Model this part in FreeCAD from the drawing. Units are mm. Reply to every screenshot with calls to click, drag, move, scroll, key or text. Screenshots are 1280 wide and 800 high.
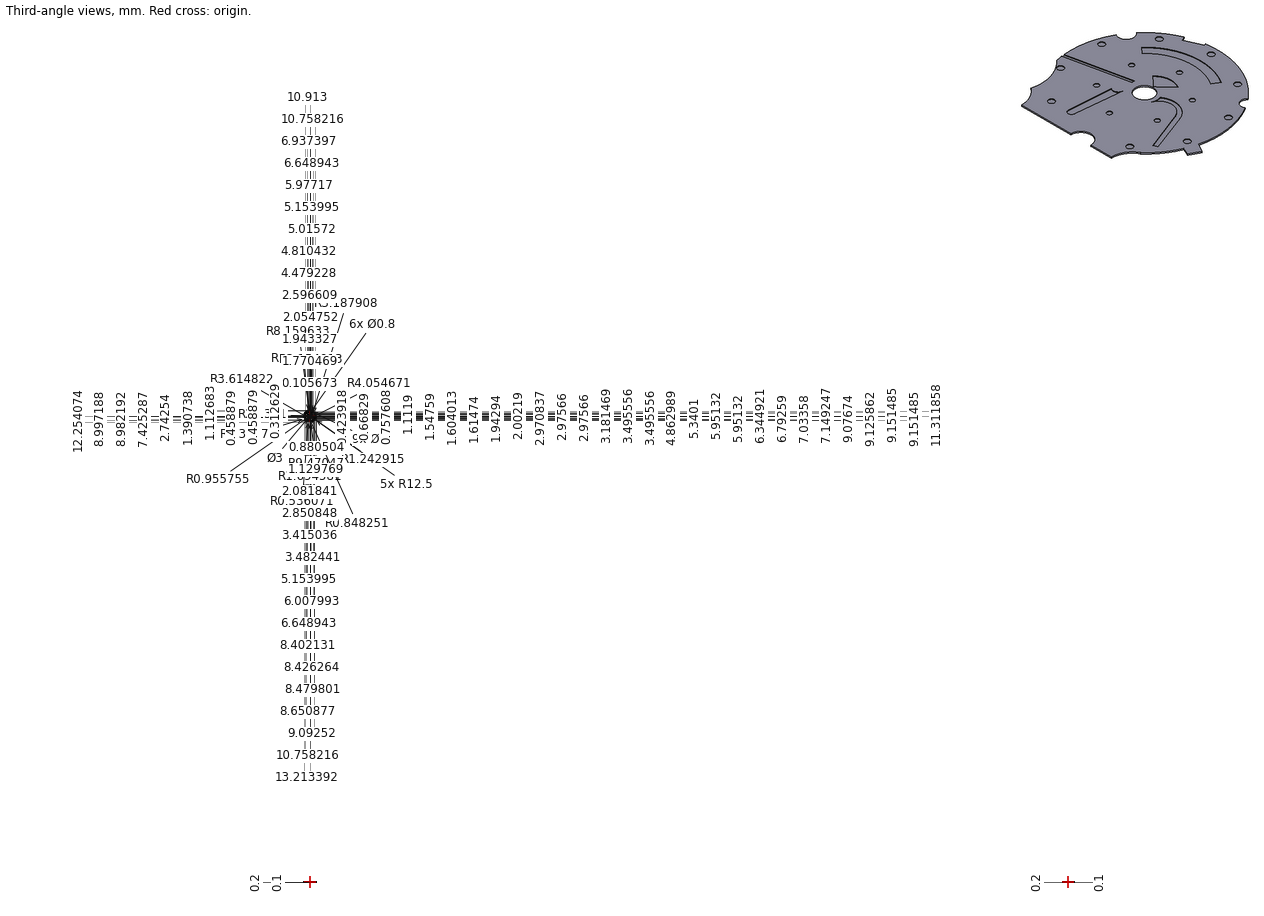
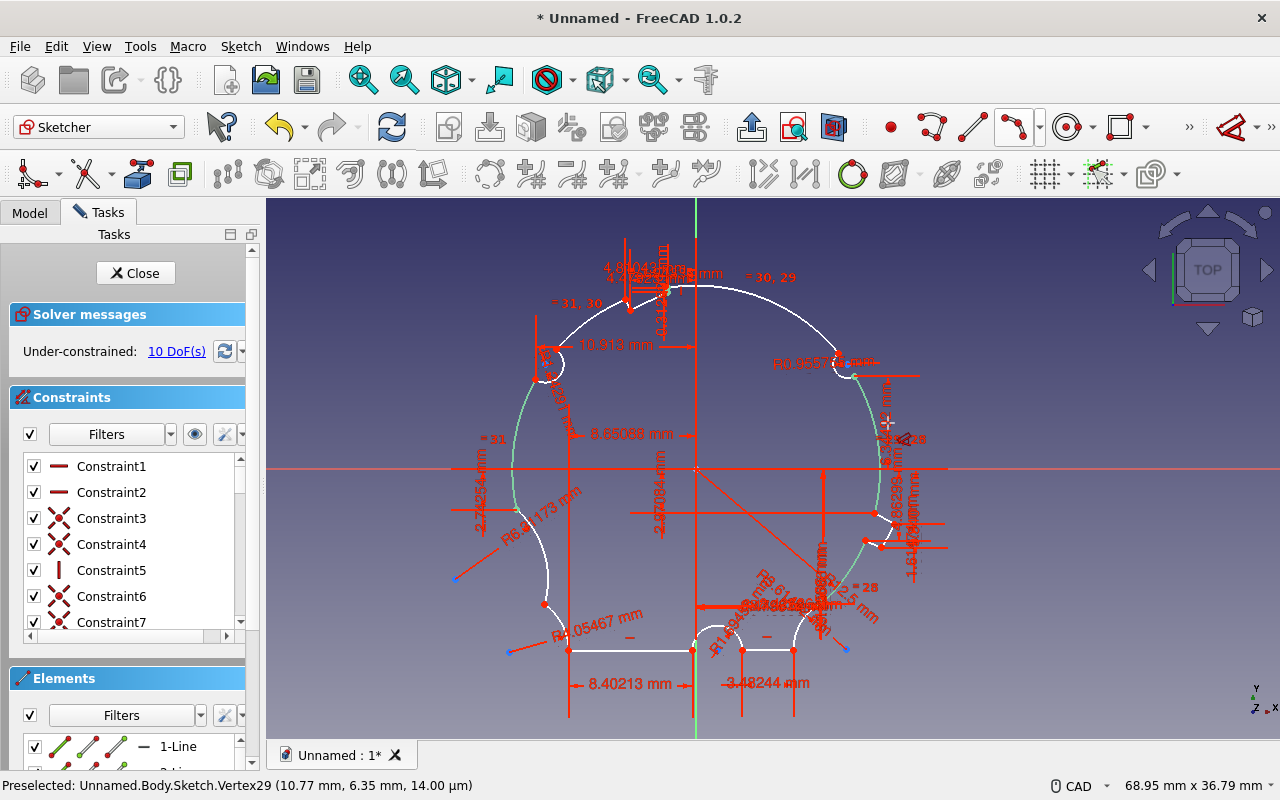
click(545, 604)
click(511, 568)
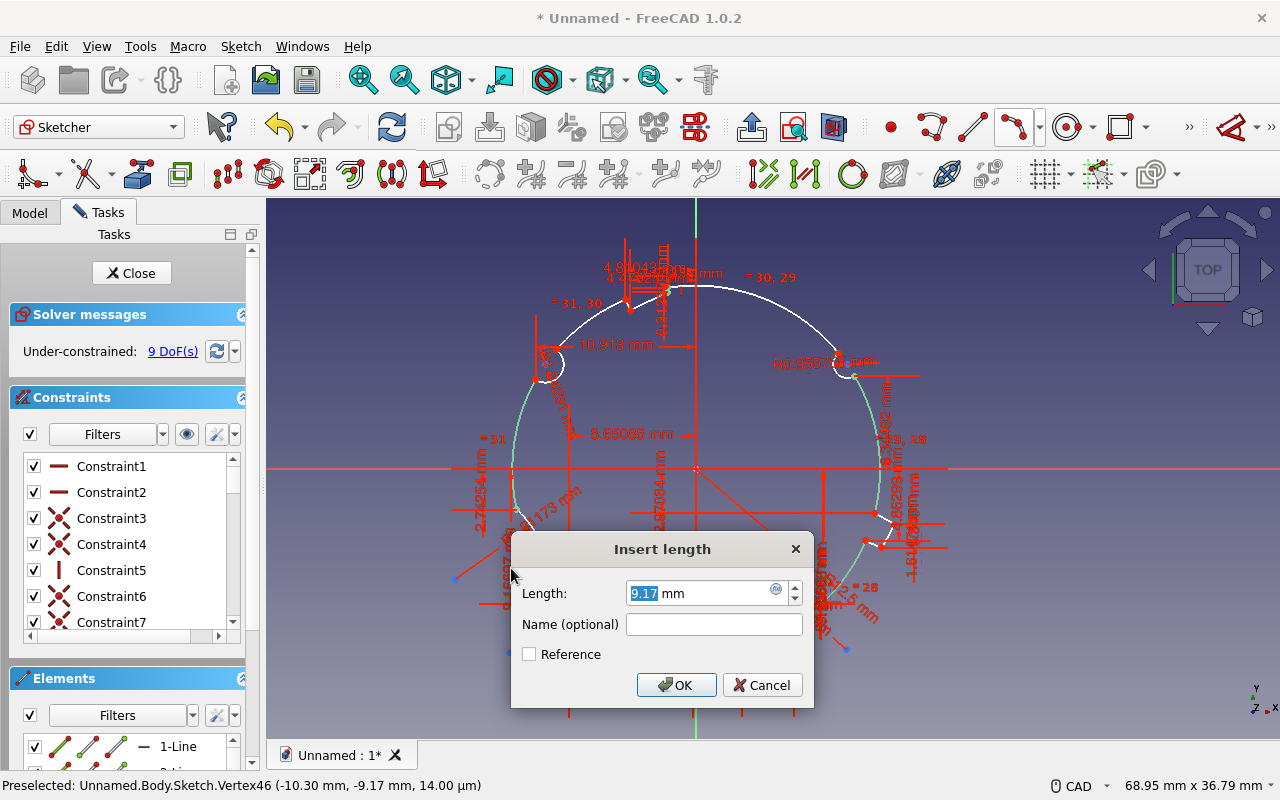
text(8.982192)
key(Return)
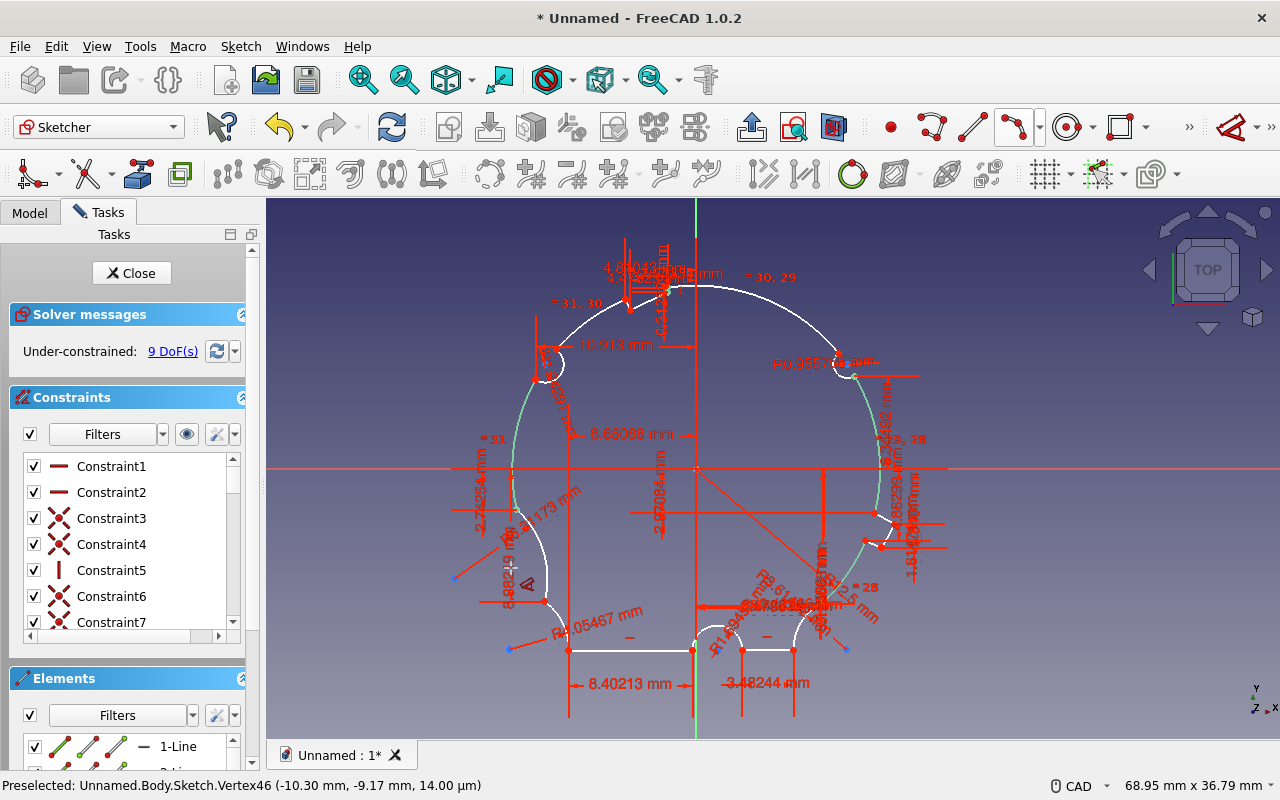
scroll(874, 544, up, 5)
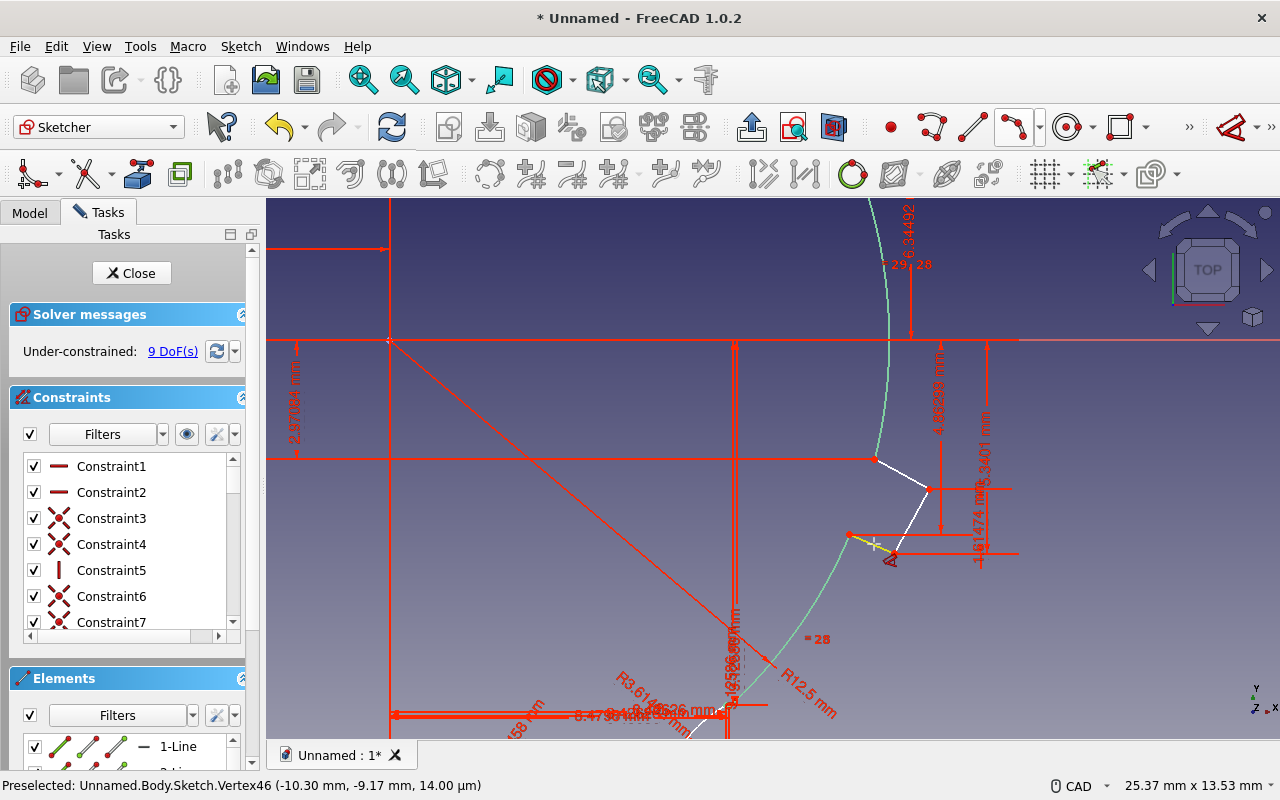
click(872, 544)
click(872, 588)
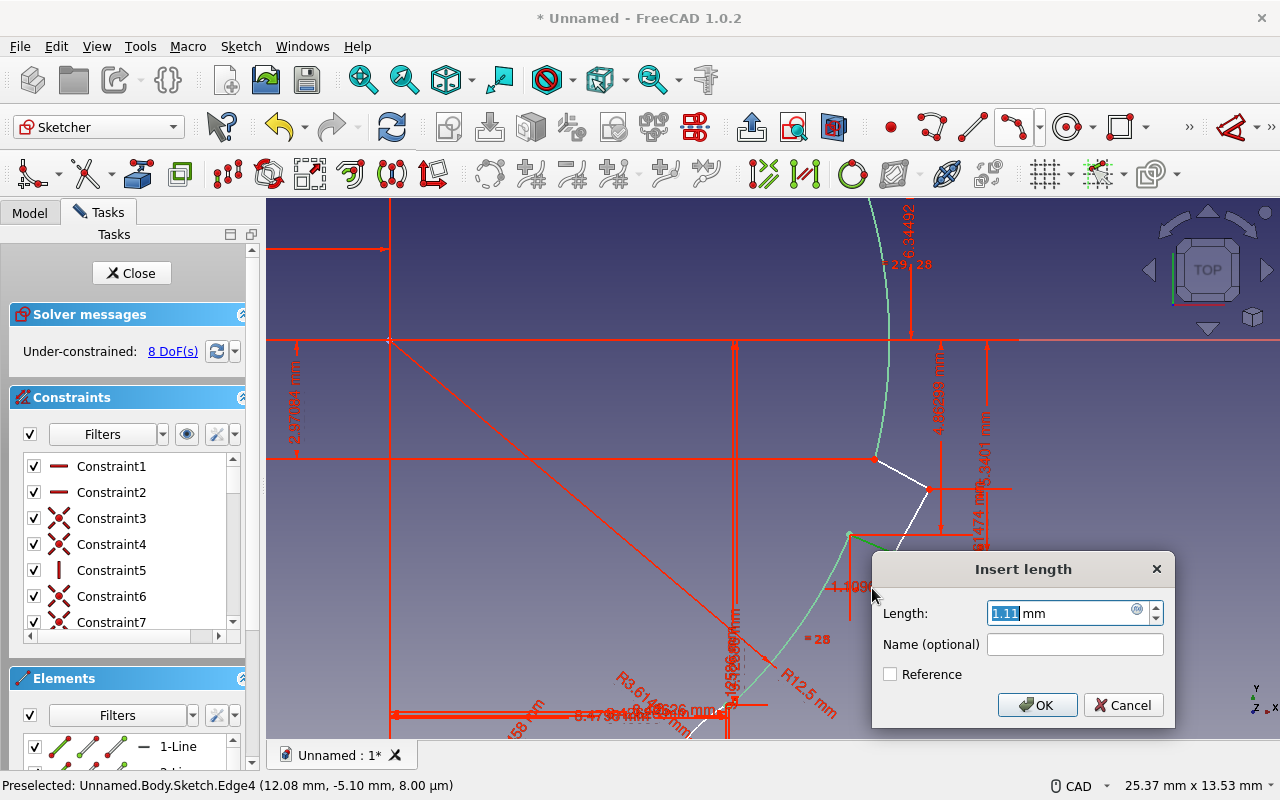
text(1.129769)
key(Return)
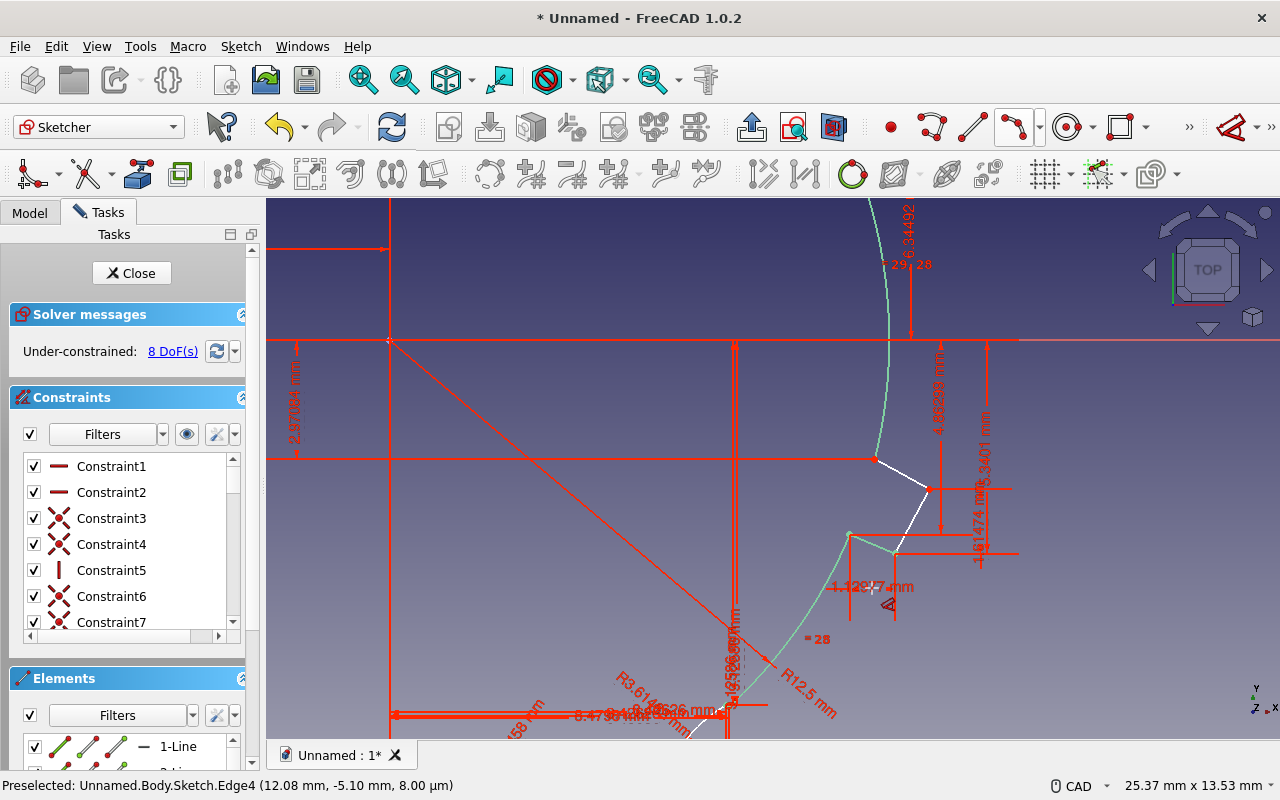
click(905, 534)
click(912, 455)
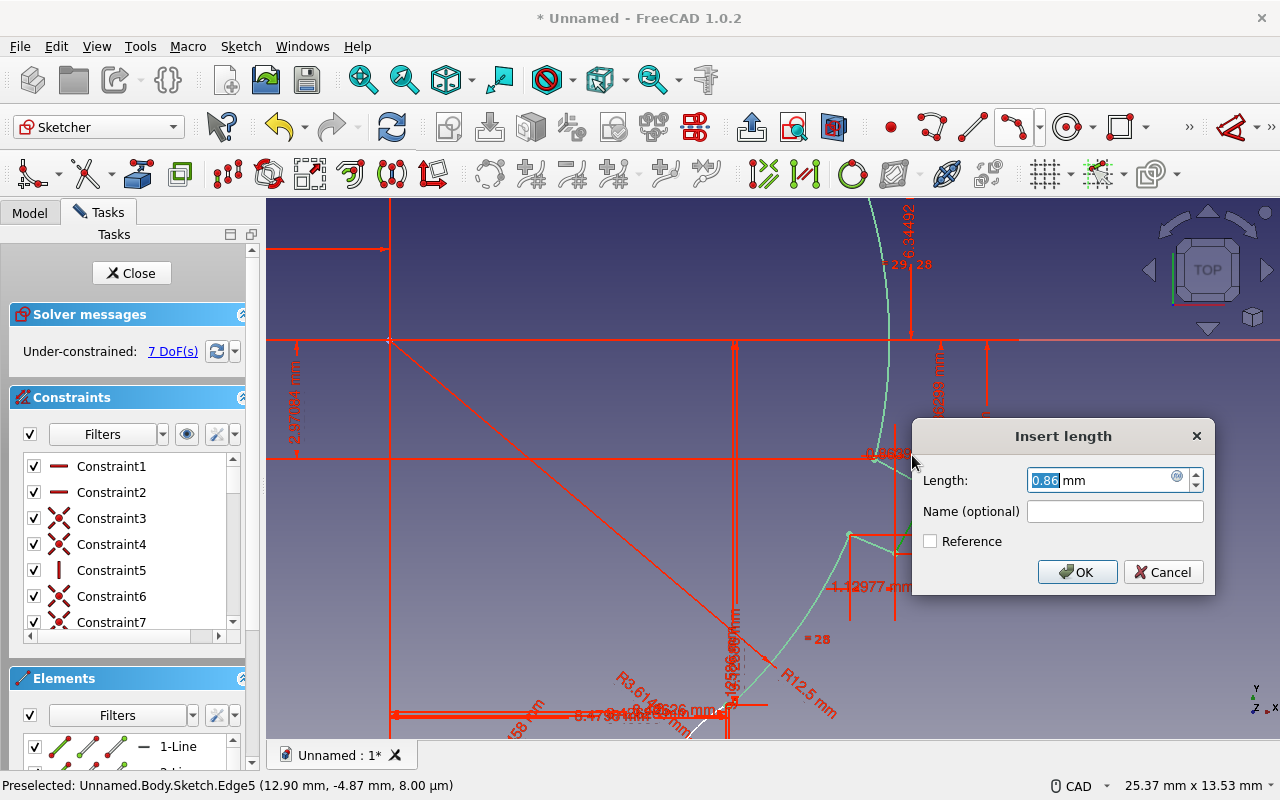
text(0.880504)
key(Return)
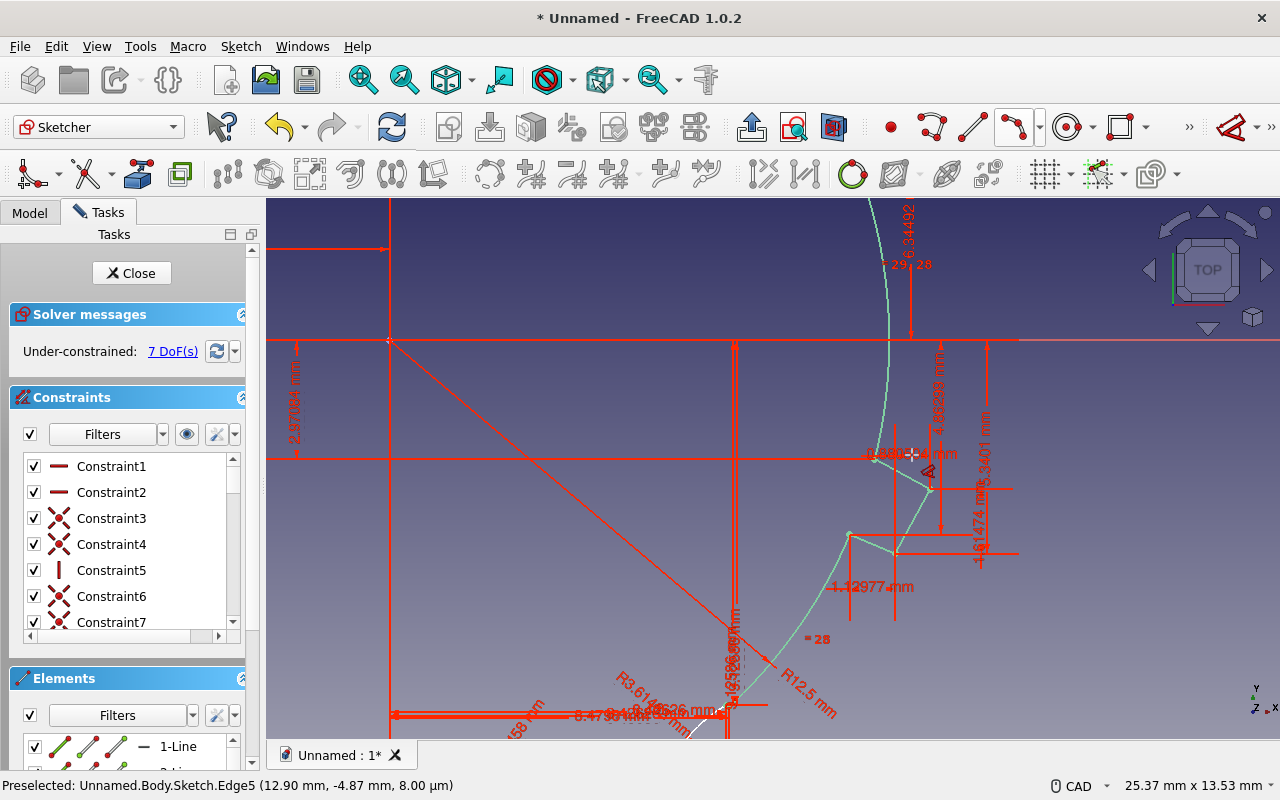
scroll(874, 544, down, 5)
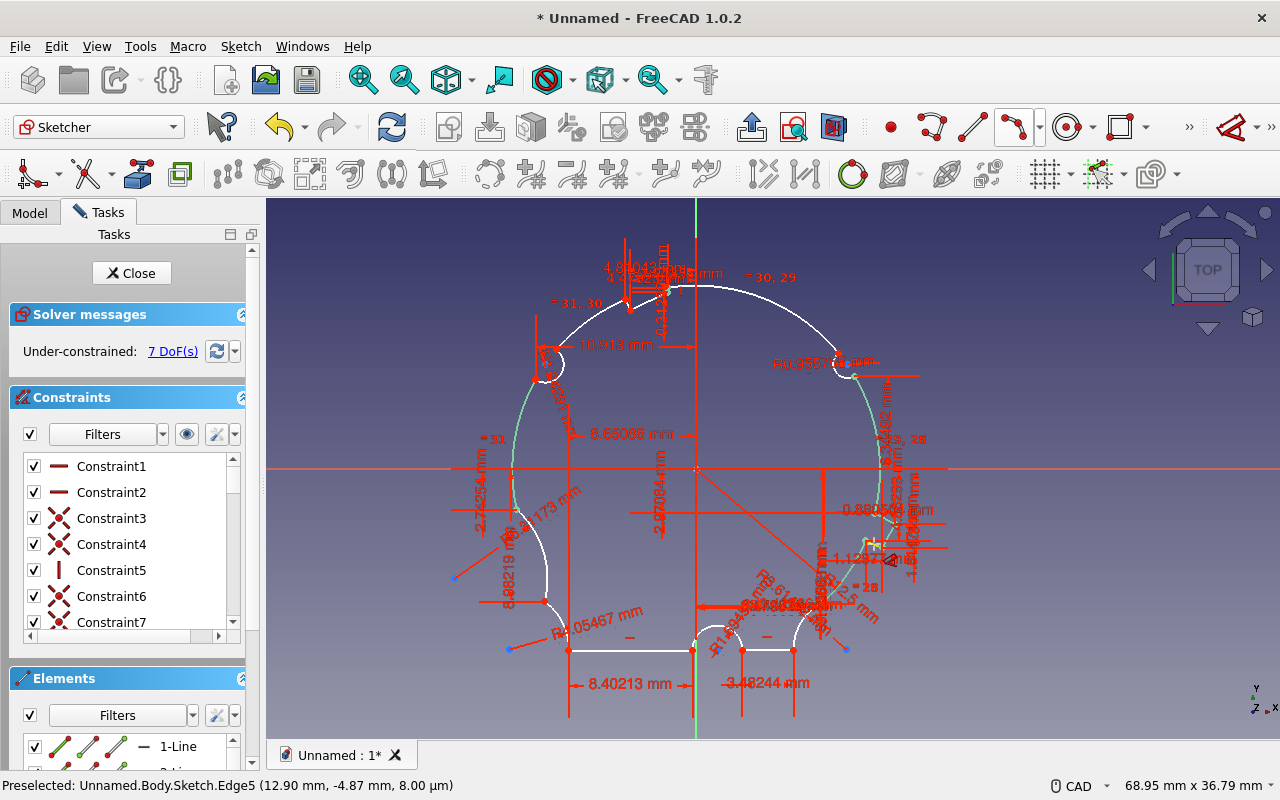
scroll(656, 298, up, 5)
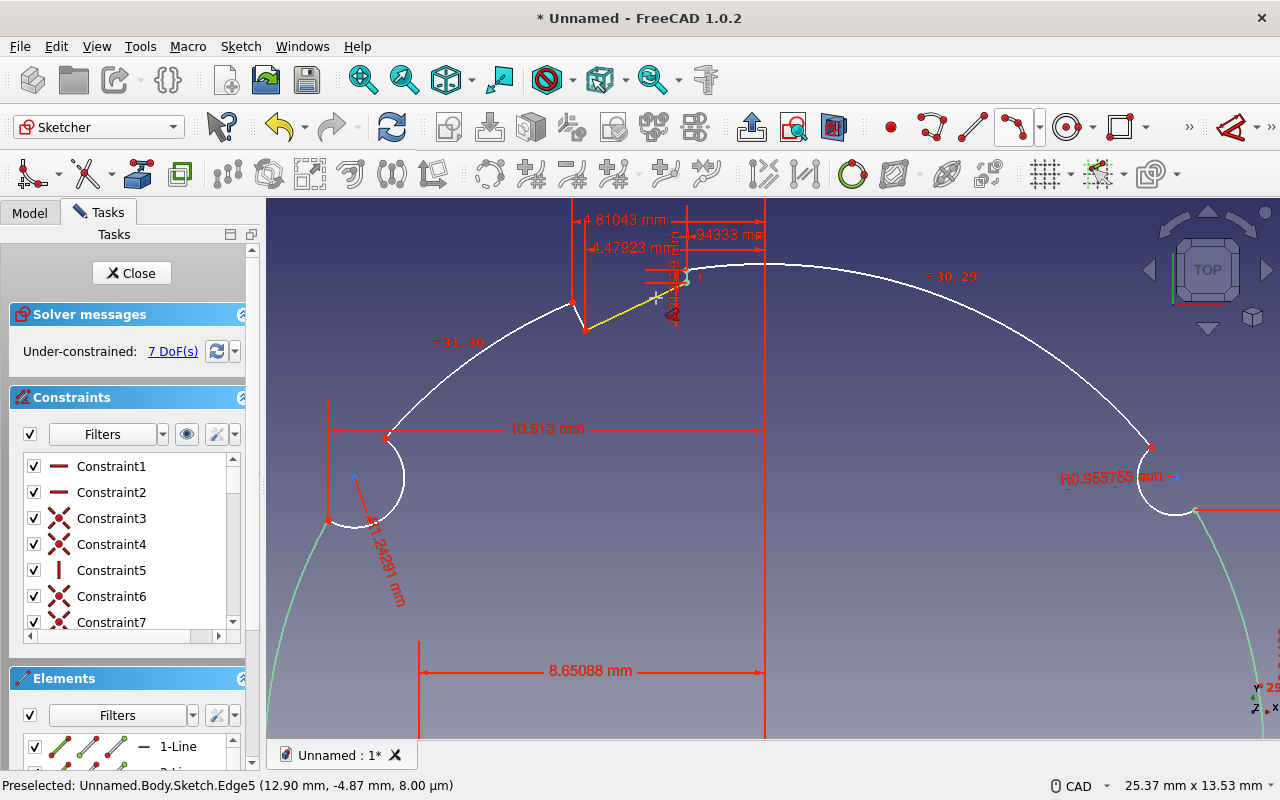
click(656, 297)
click(551, 296)